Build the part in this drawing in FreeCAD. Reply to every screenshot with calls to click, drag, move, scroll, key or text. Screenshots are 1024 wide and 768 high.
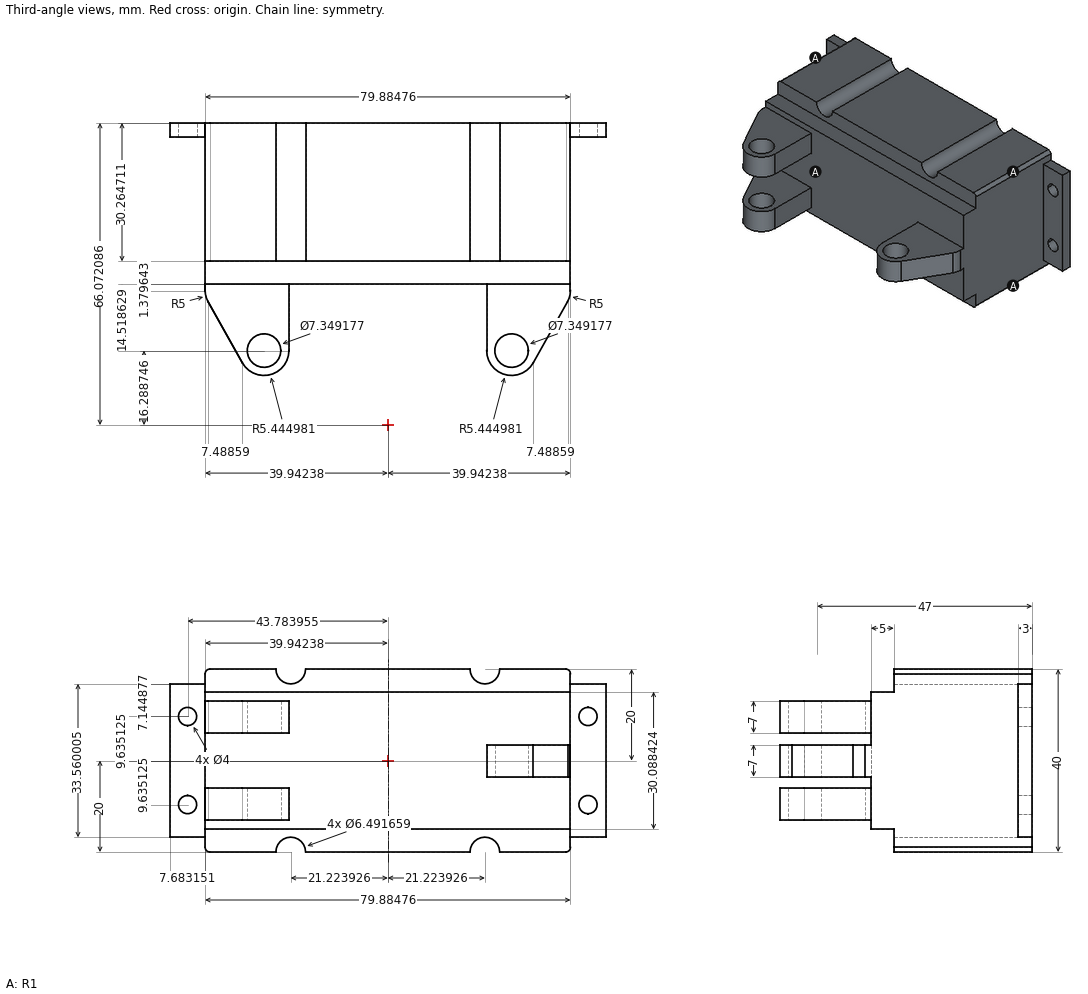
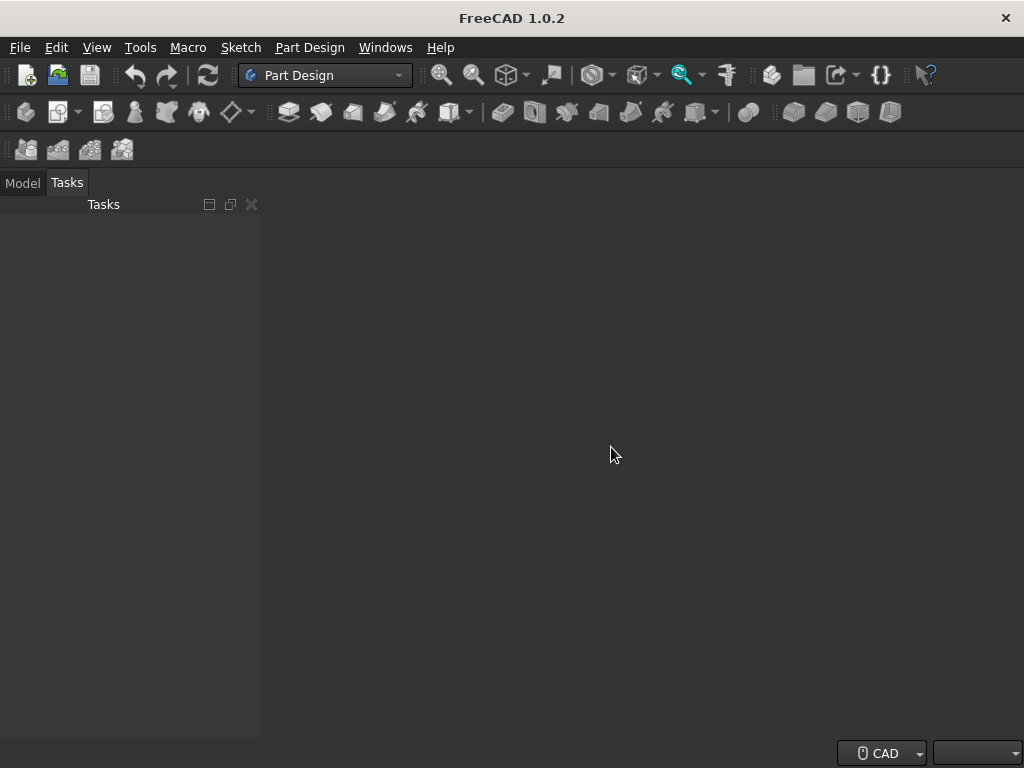
click(26, 76)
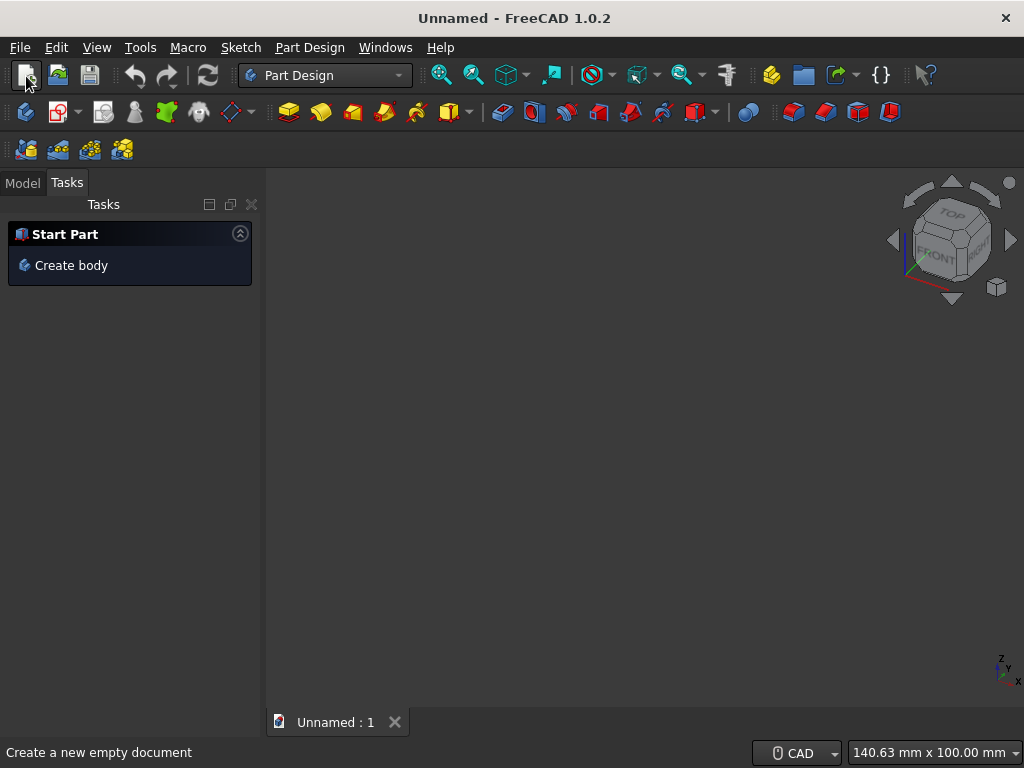
click(58, 112)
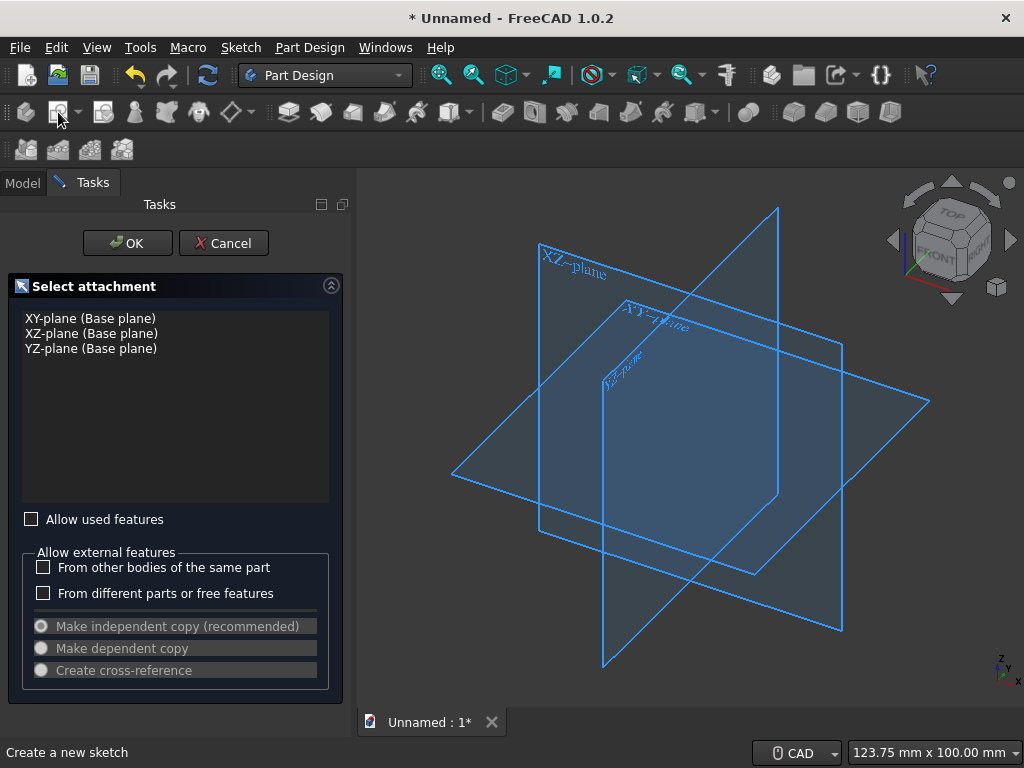
click(82, 318)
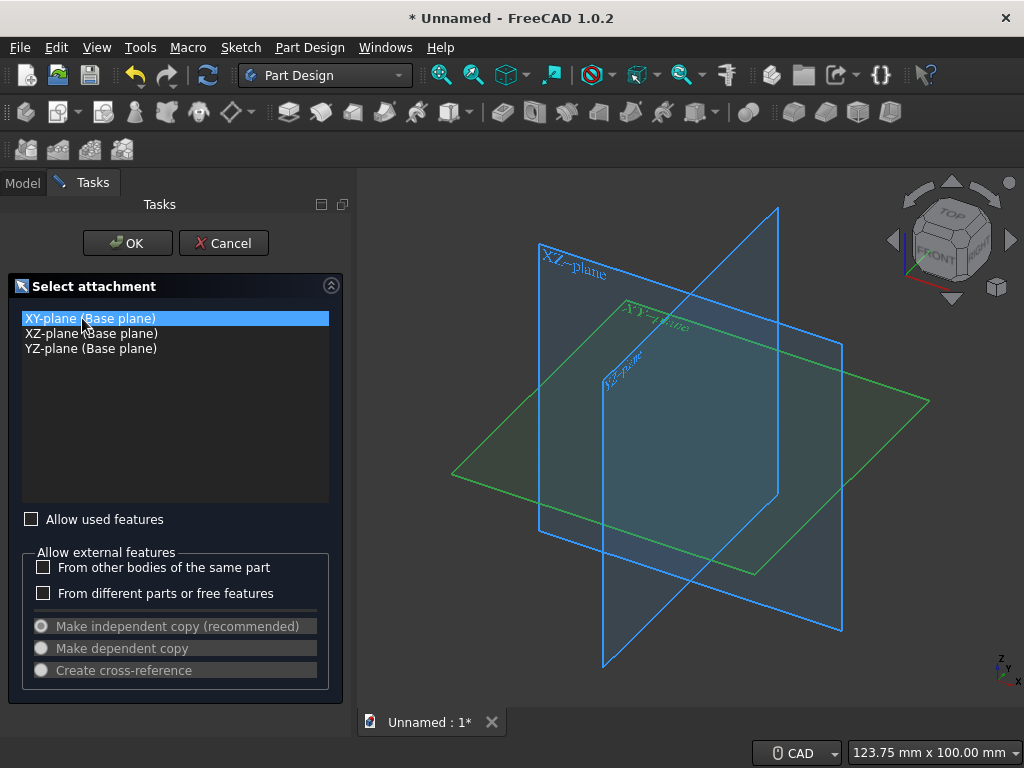
click(128, 243)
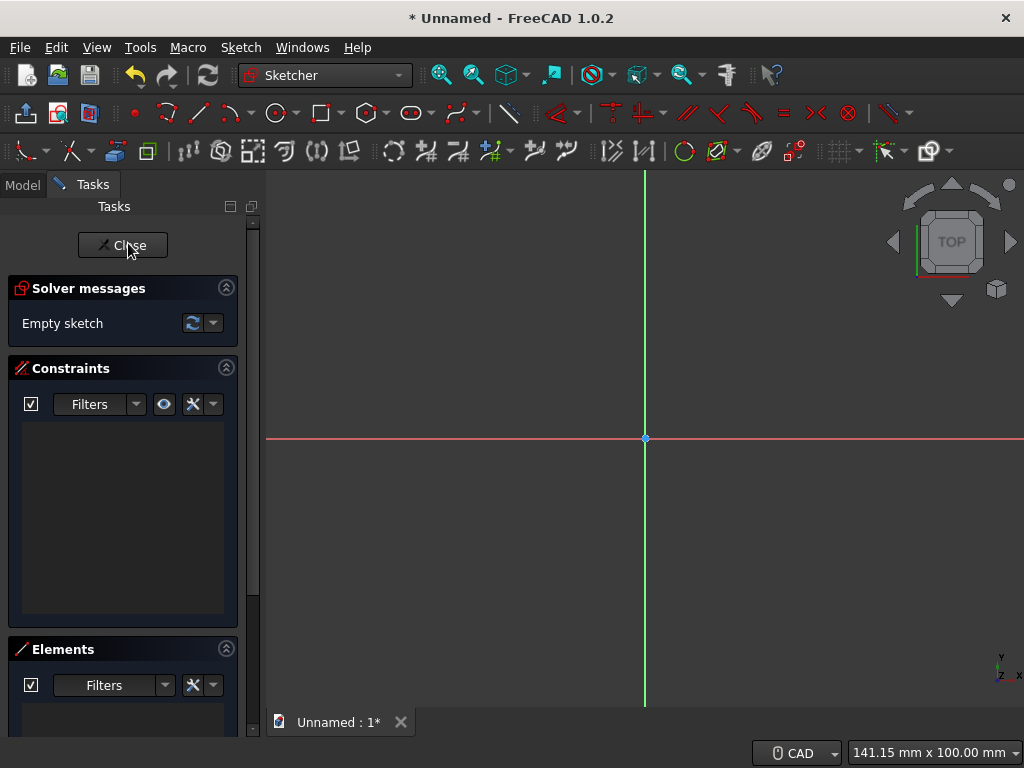
scroll(437, 679, down, 2)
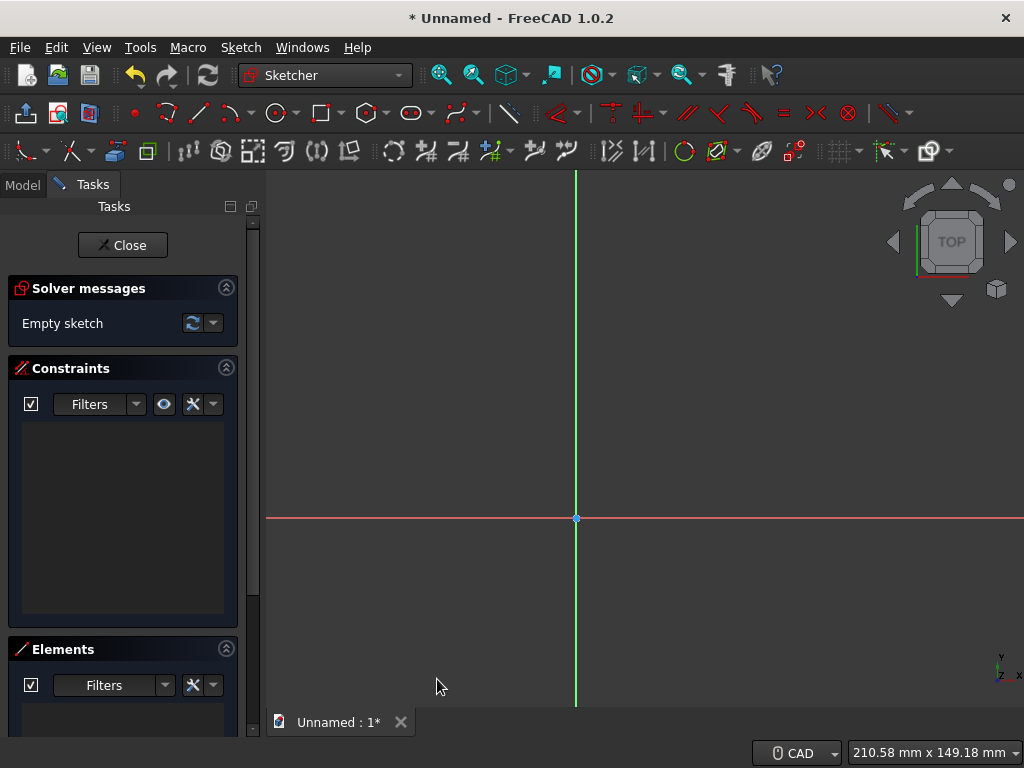
scroll(577, 319, up, 2)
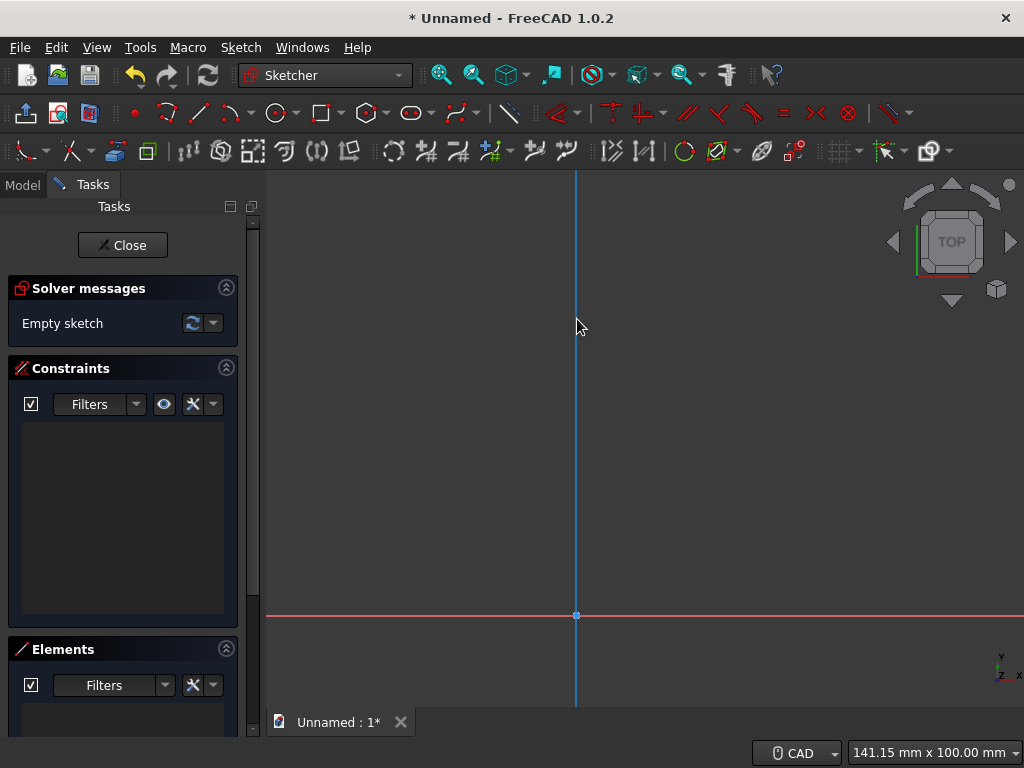
key(g)
key(r)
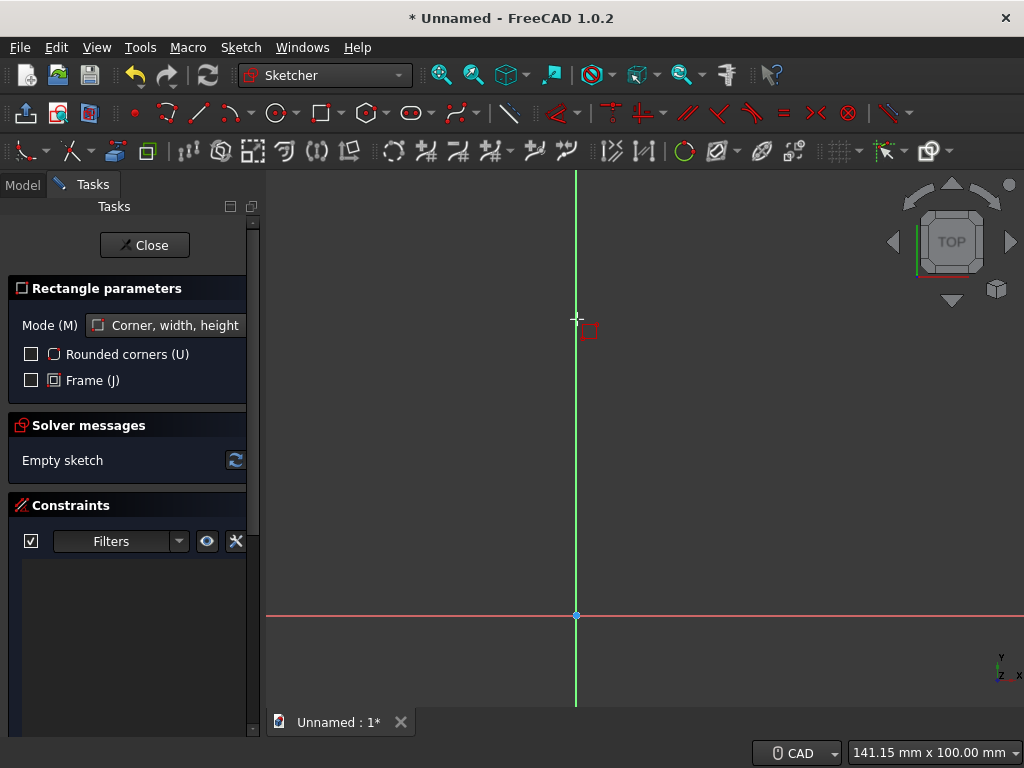
click(362, 261)
click(791, 424)
key(Escape)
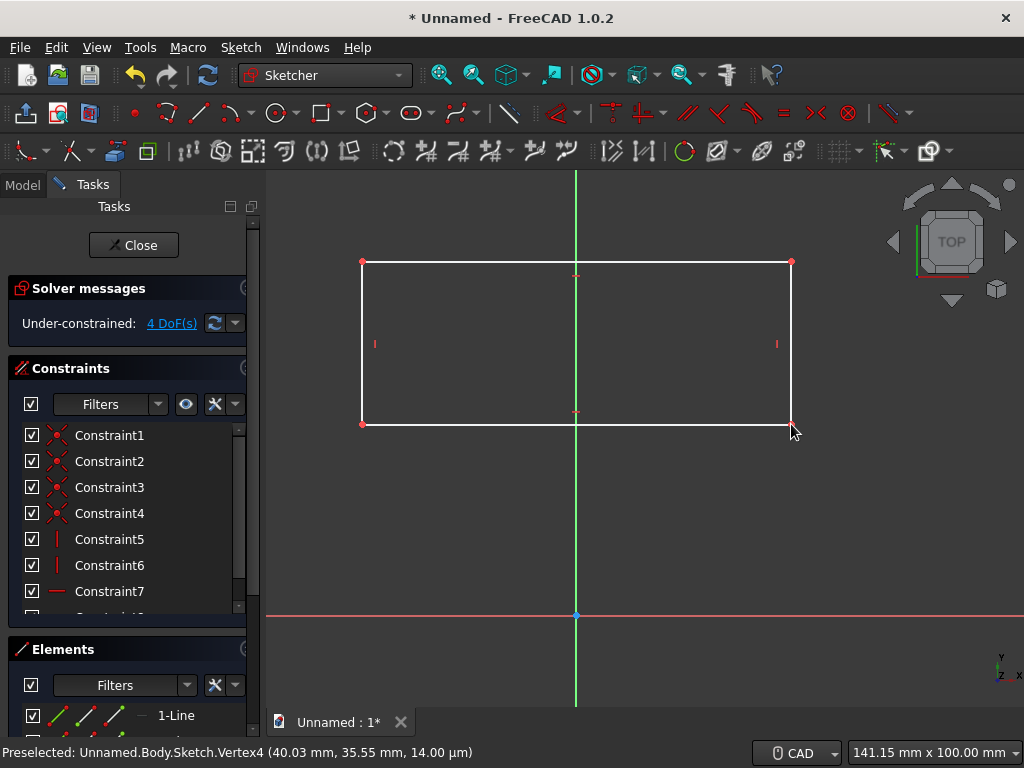
key(d)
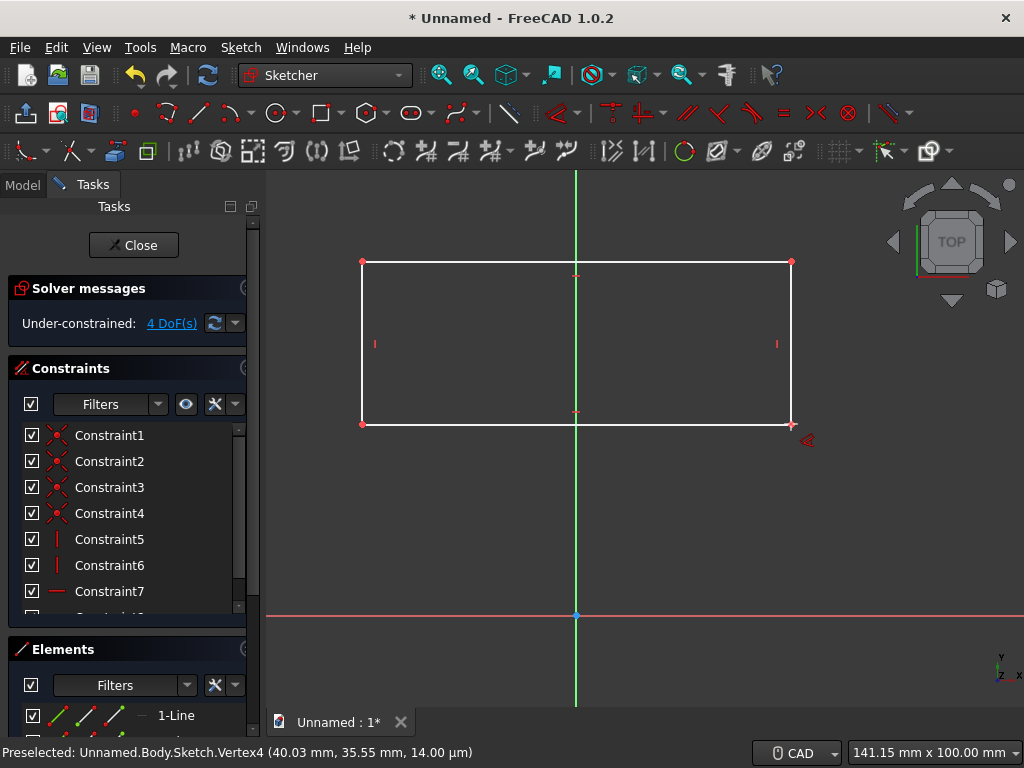
click(491, 425)
click(478, 391)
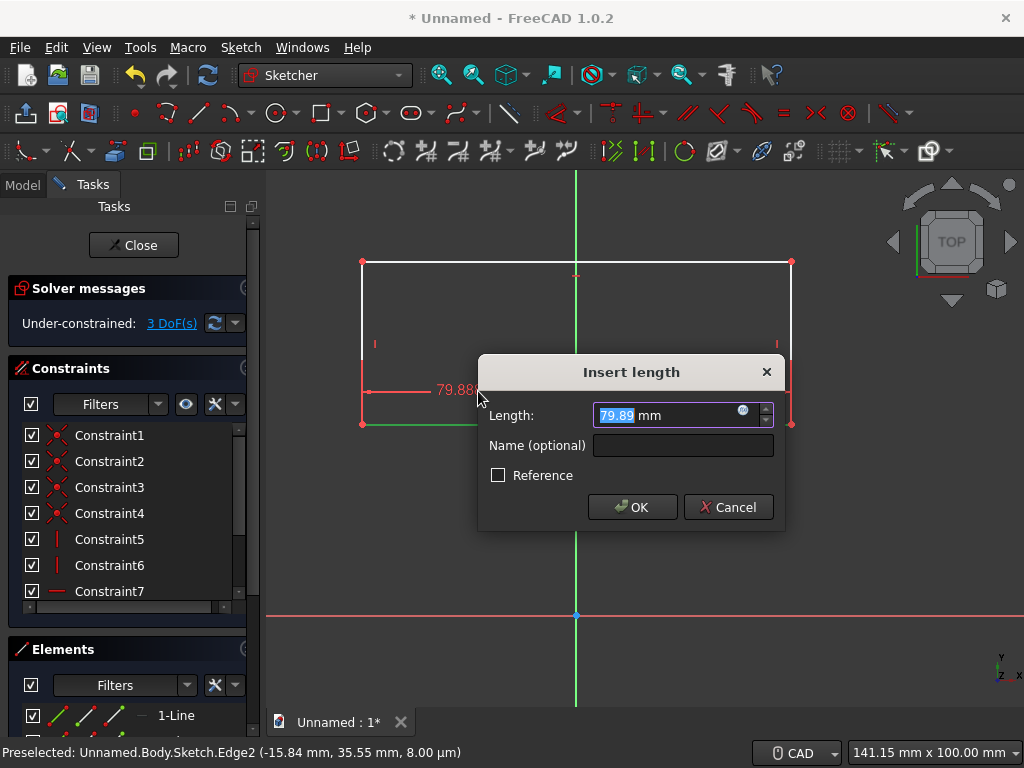
text(79.88476)
key(Return)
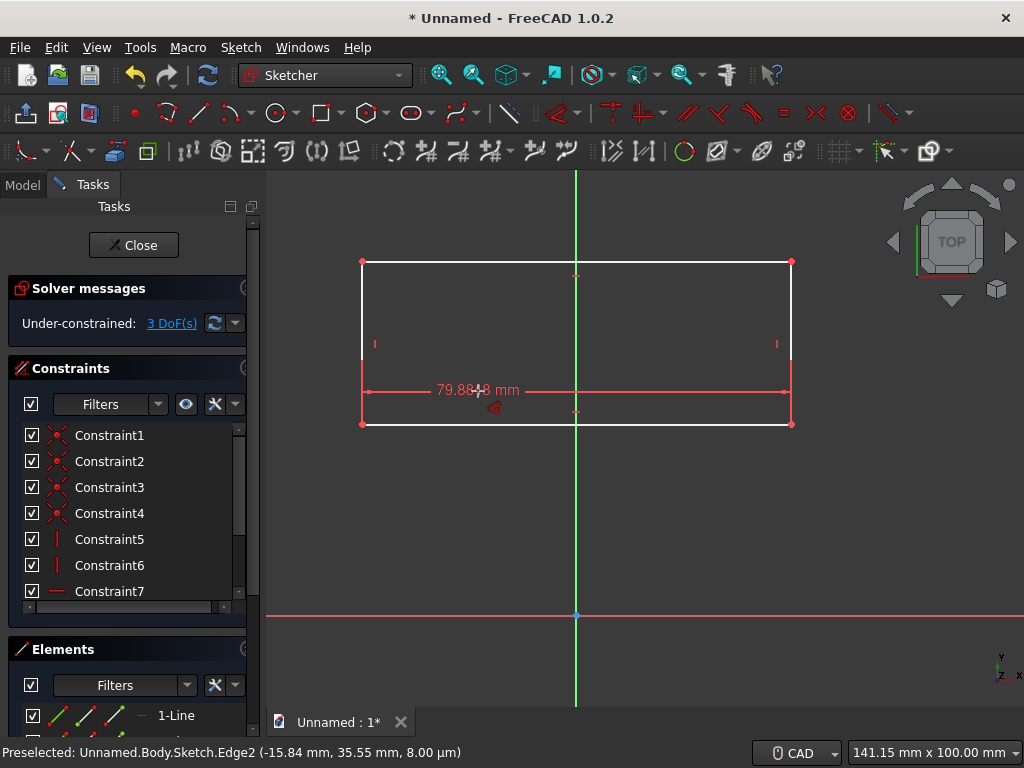
click(362, 311)
click(328, 343)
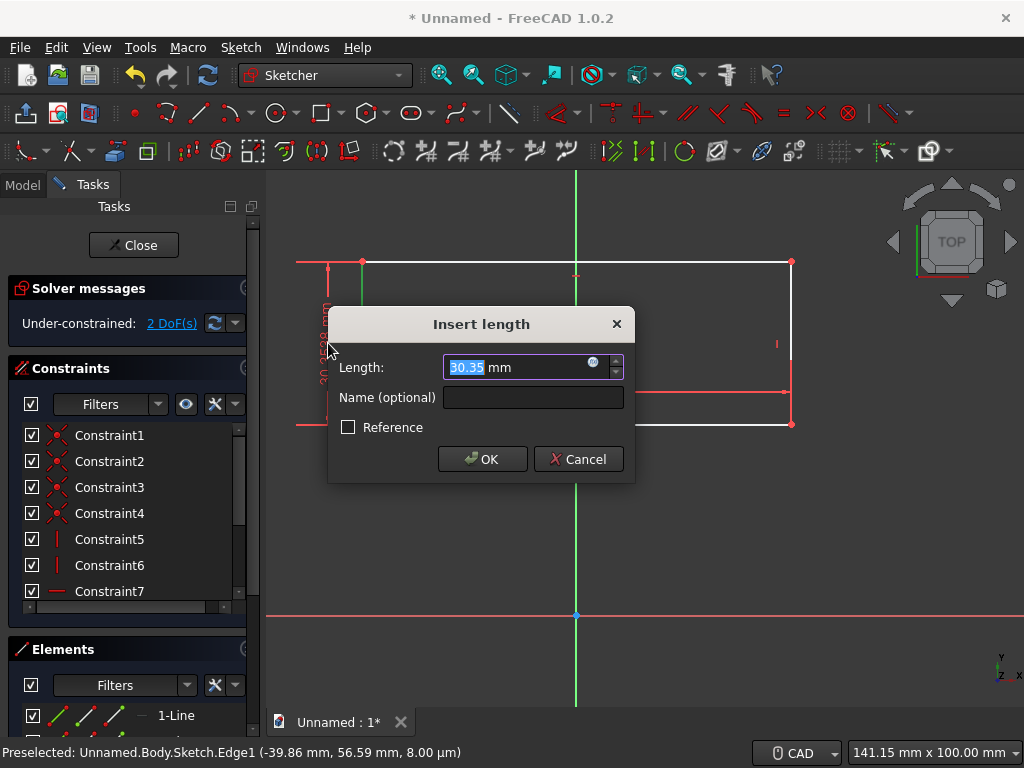
text(30.264711)
key(Return)